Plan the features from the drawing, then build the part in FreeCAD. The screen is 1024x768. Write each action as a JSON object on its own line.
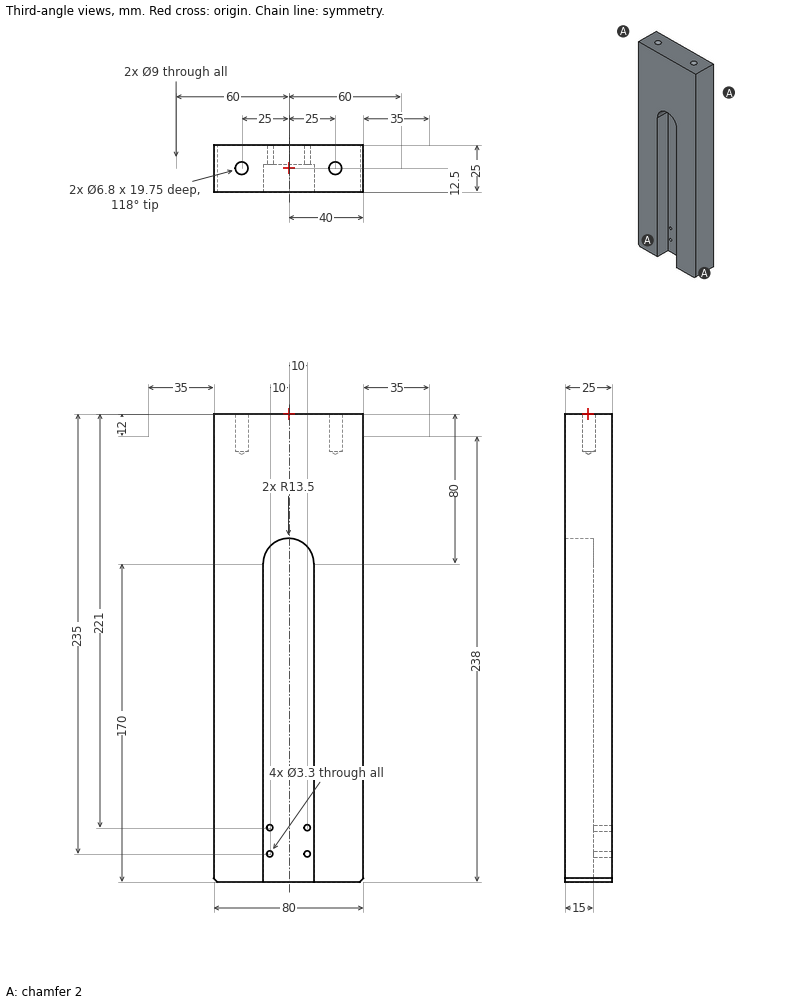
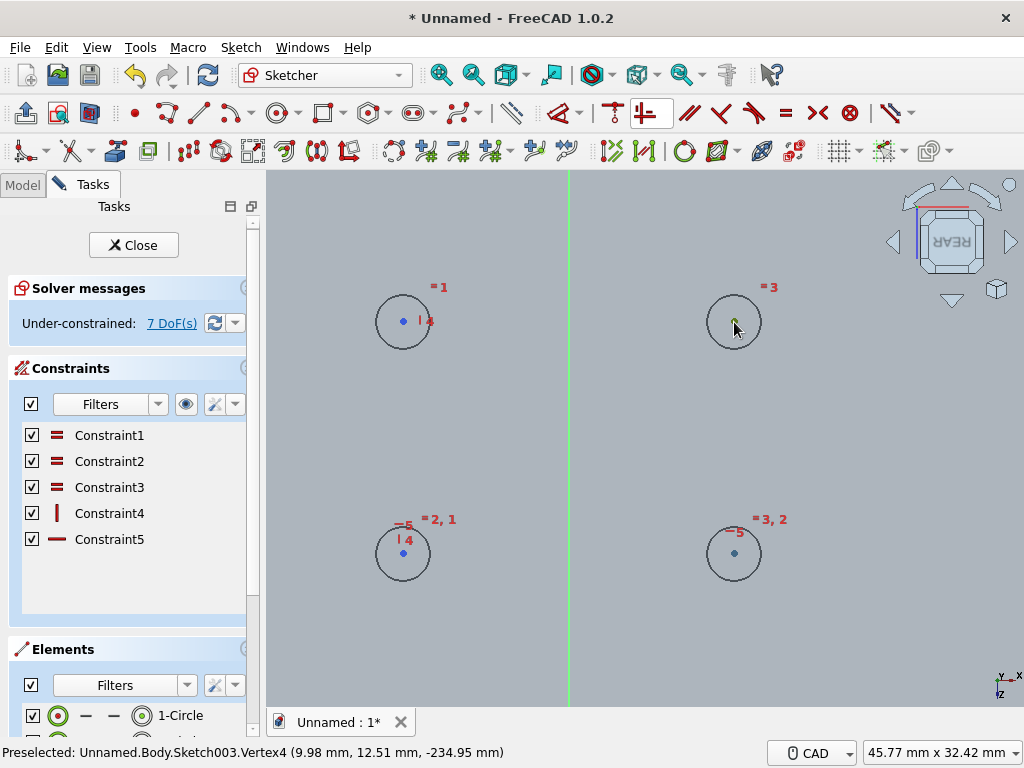
{"action": "left_click", "coordinate": [668, 114]}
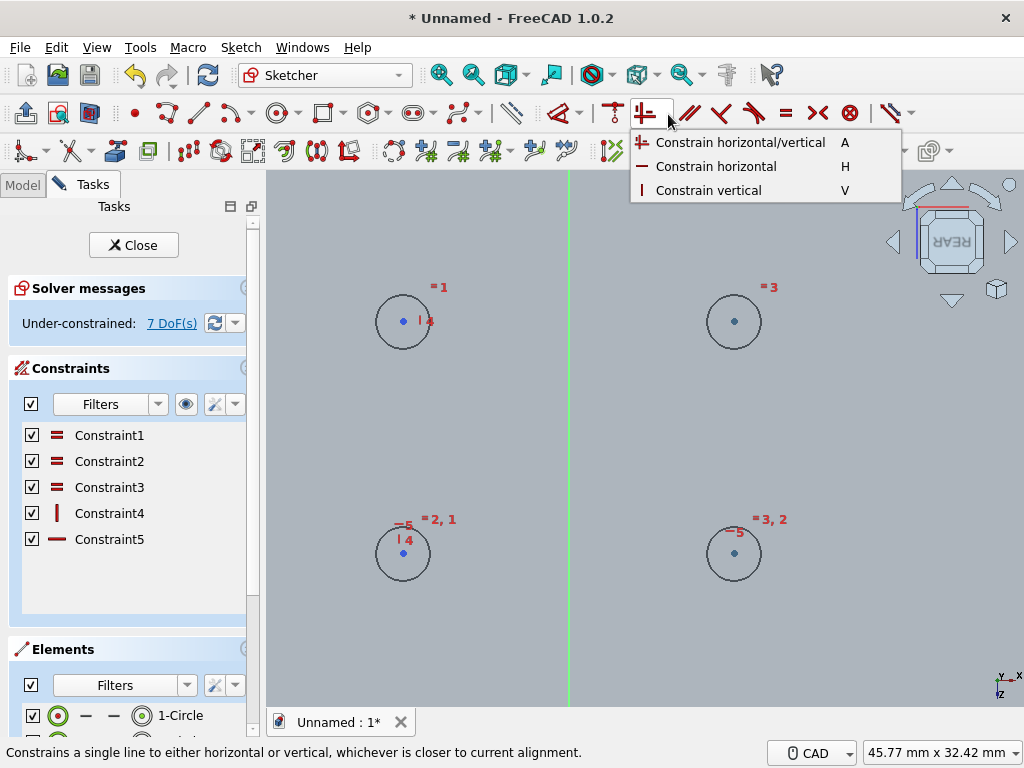
{"action": "left_click", "coordinate": [766, 190]}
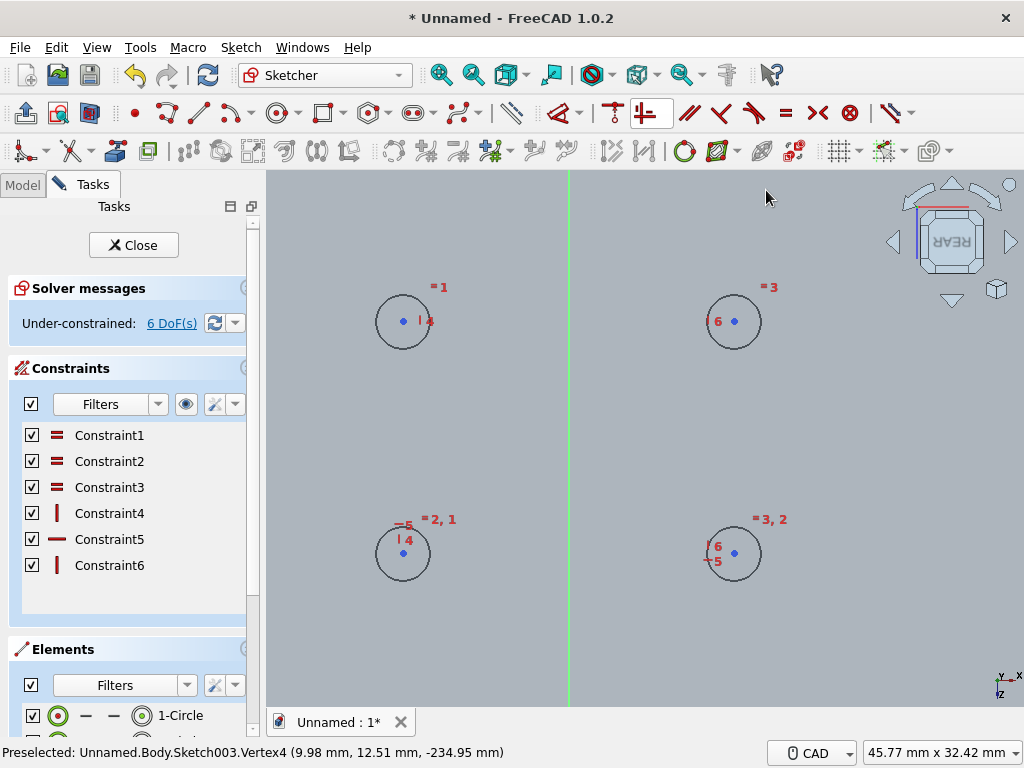
{"action": "left_click", "coordinate": [403, 322]}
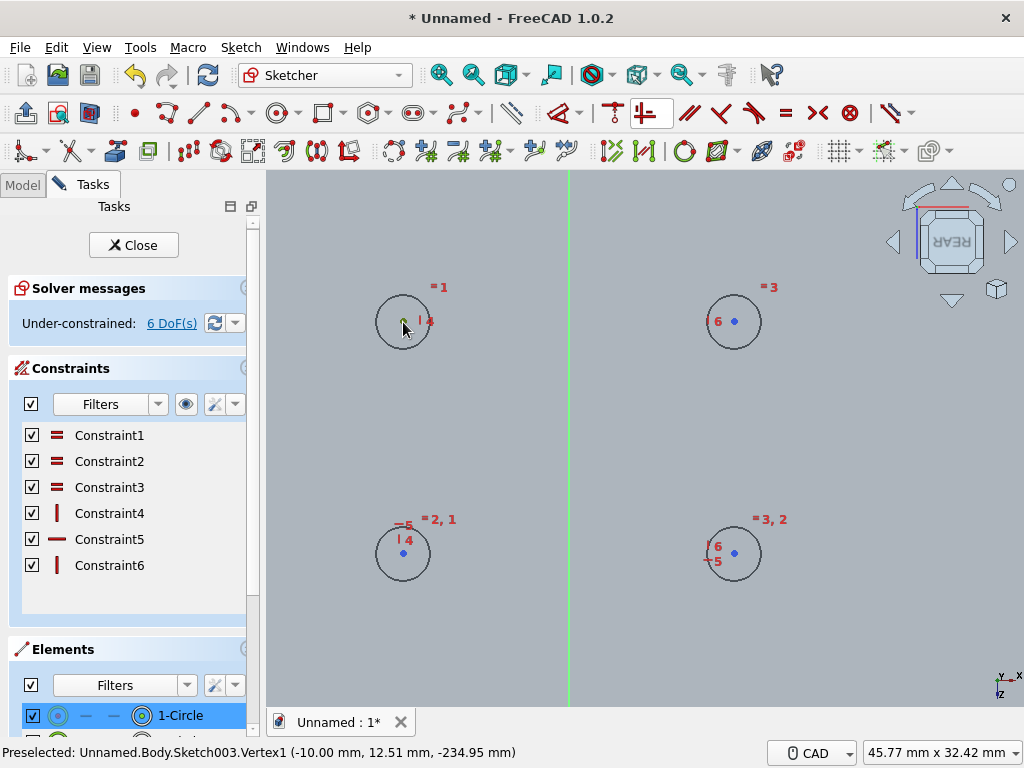
{"action": "left_click", "coordinate": [734, 322]}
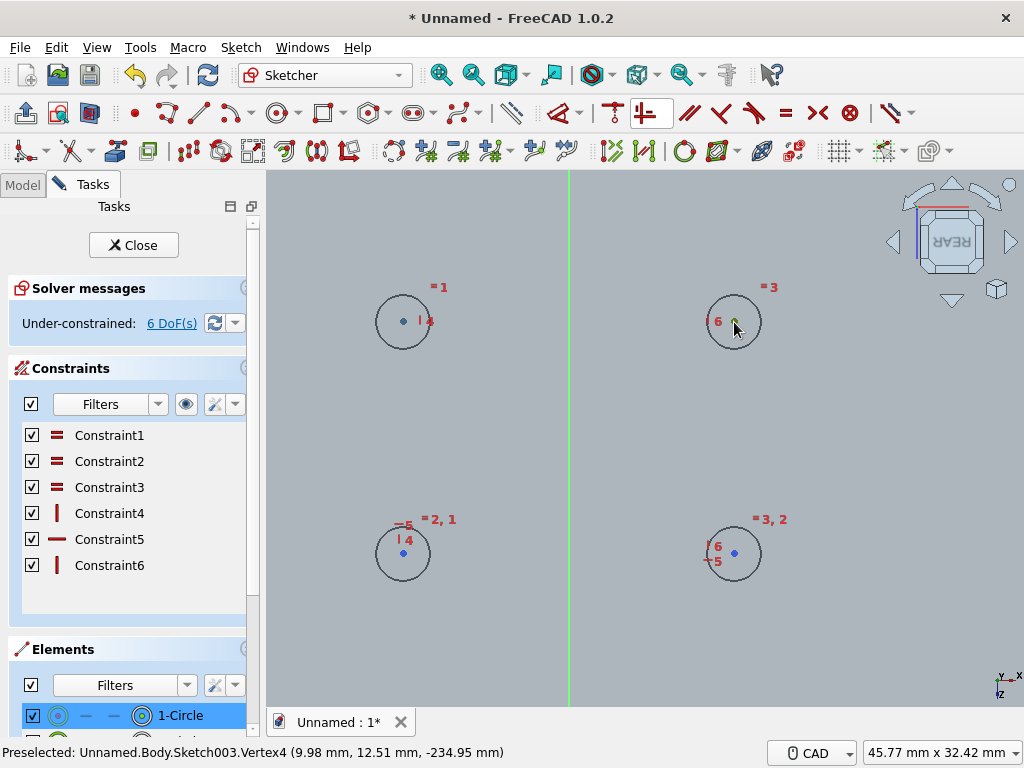
{"action": "left_click", "coordinate": [668, 114]}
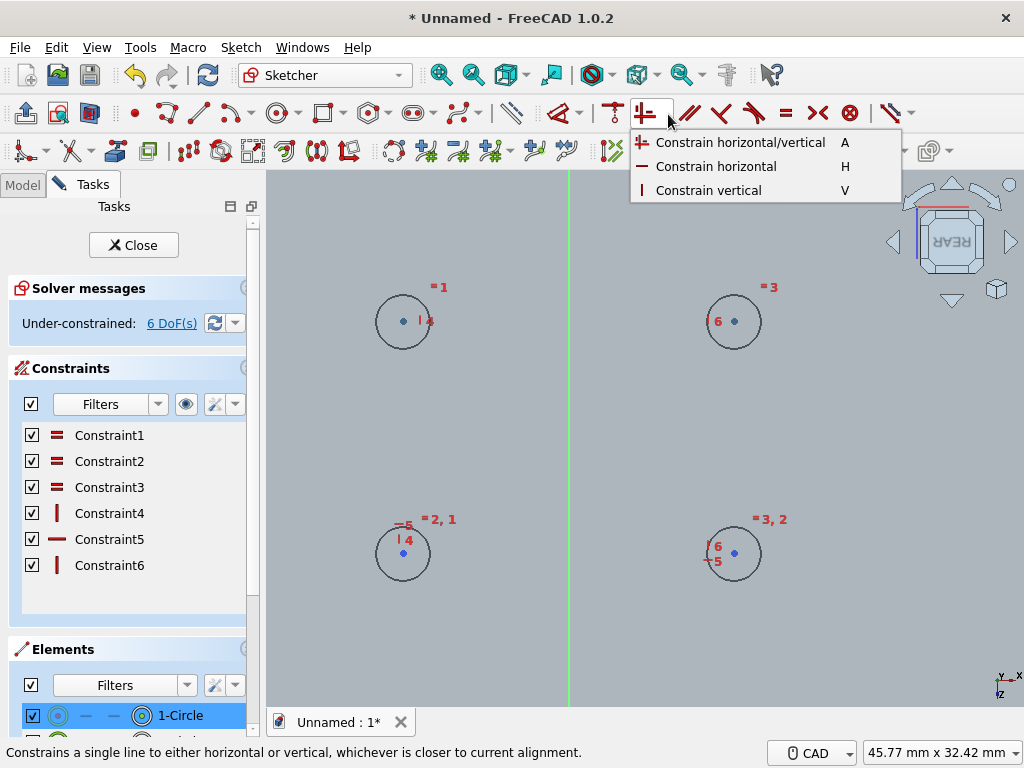
{"action": "left_click", "coordinate": [766, 166]}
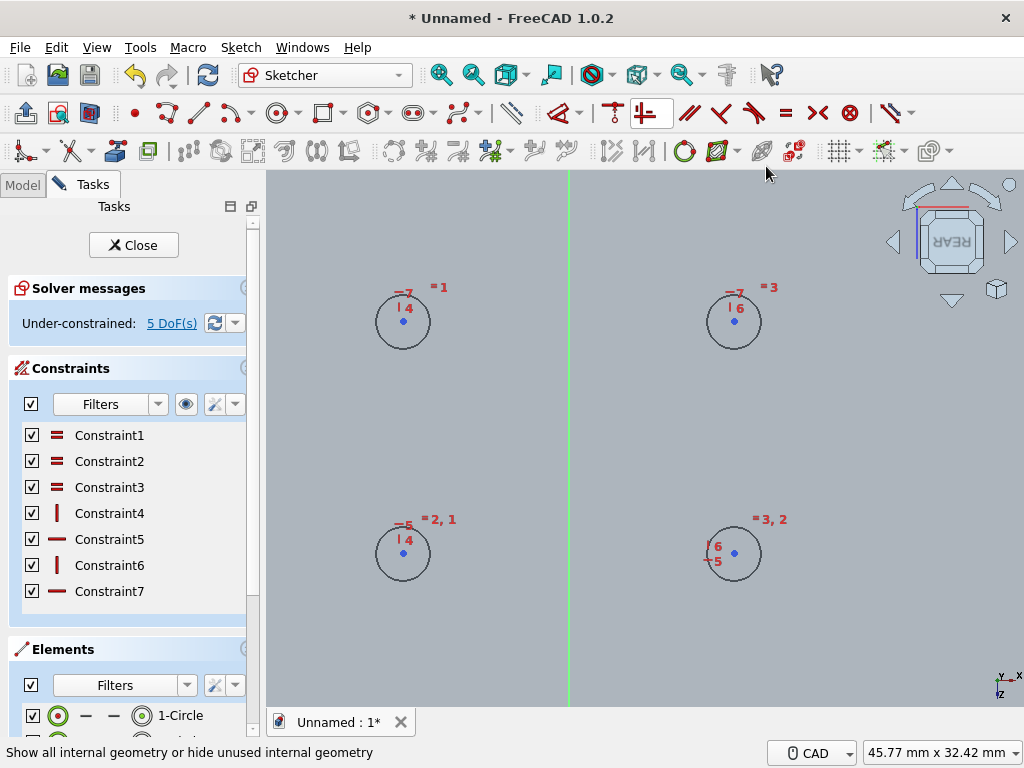
{"action": "left_click", "coordinate": [558, 114]}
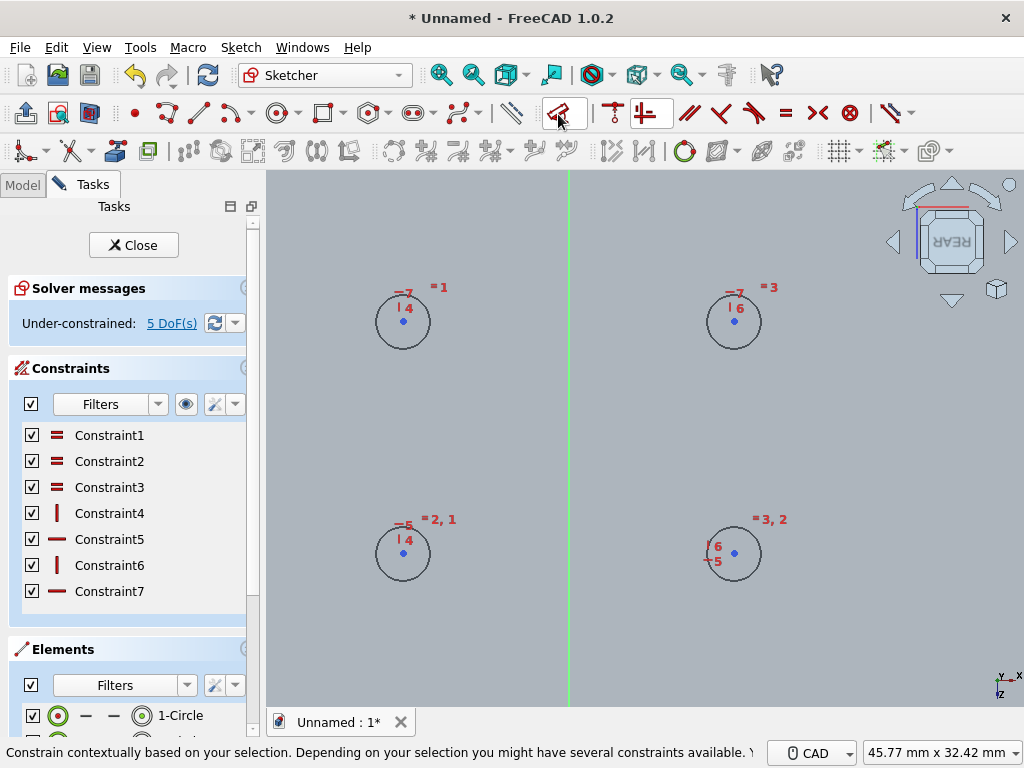
{"action": "left_click", "coordinate": [422, 303]}
{"action": "left_click", "coordinate": [445, 280]}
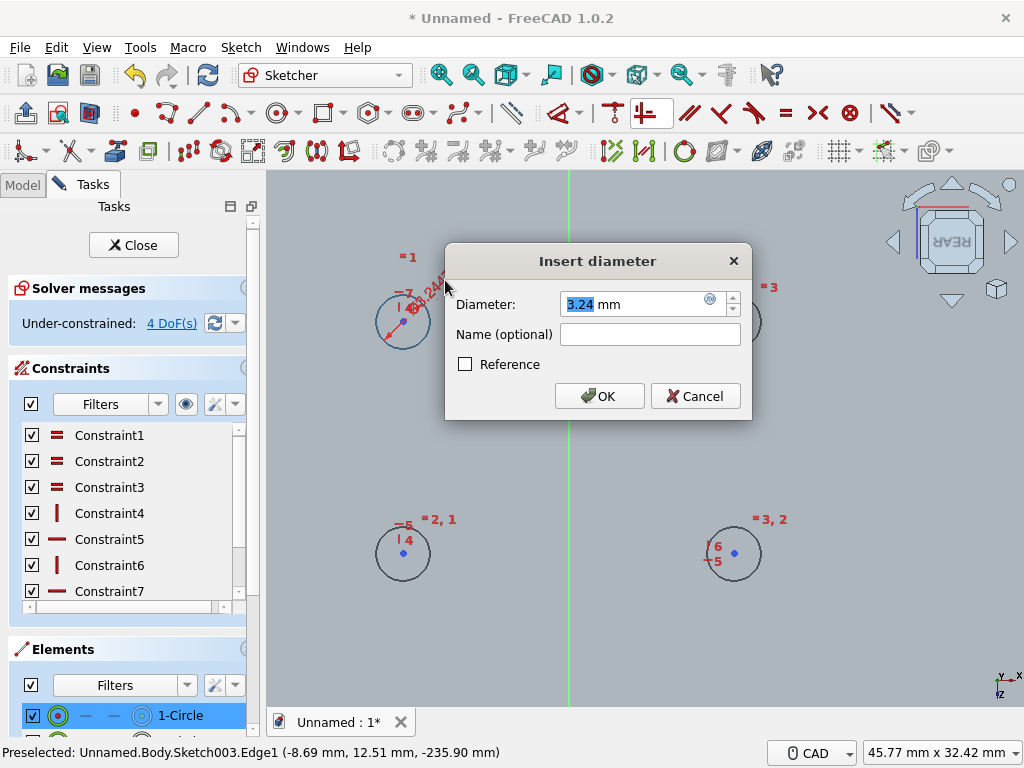
{"action": "type", "text": "3.3"}
{"action": "key", "text": "Return"}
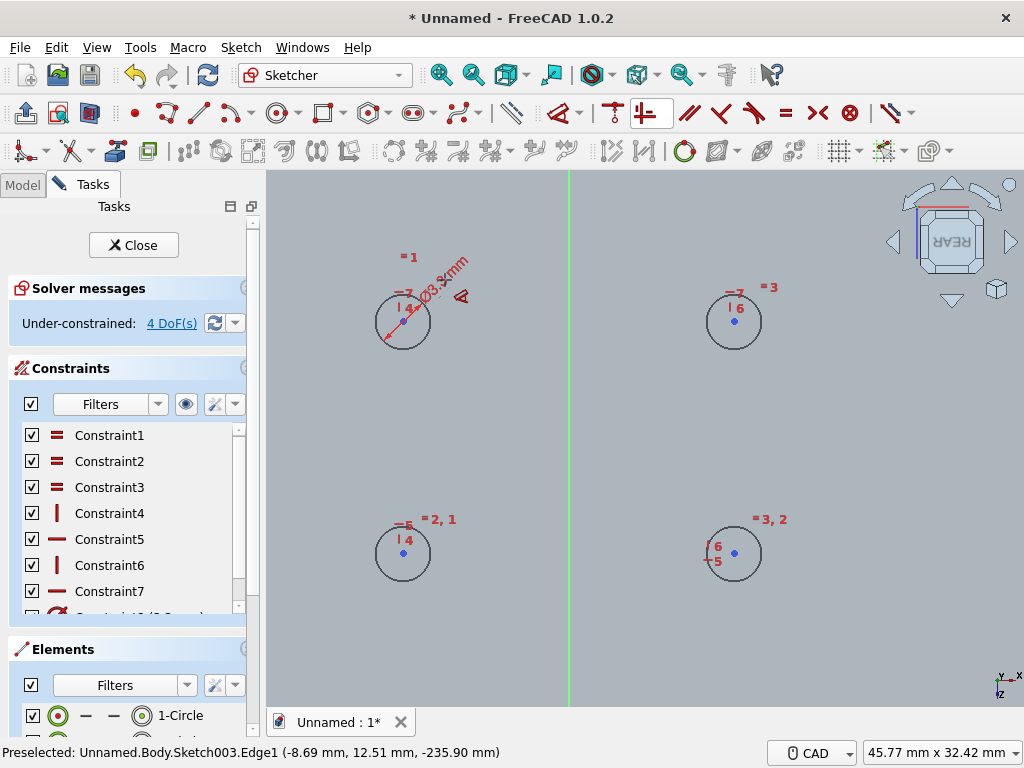
{"action": "left_click", "coordinate": [403, 322]}
{"action": "left_click", "coordinate": [524, 288]}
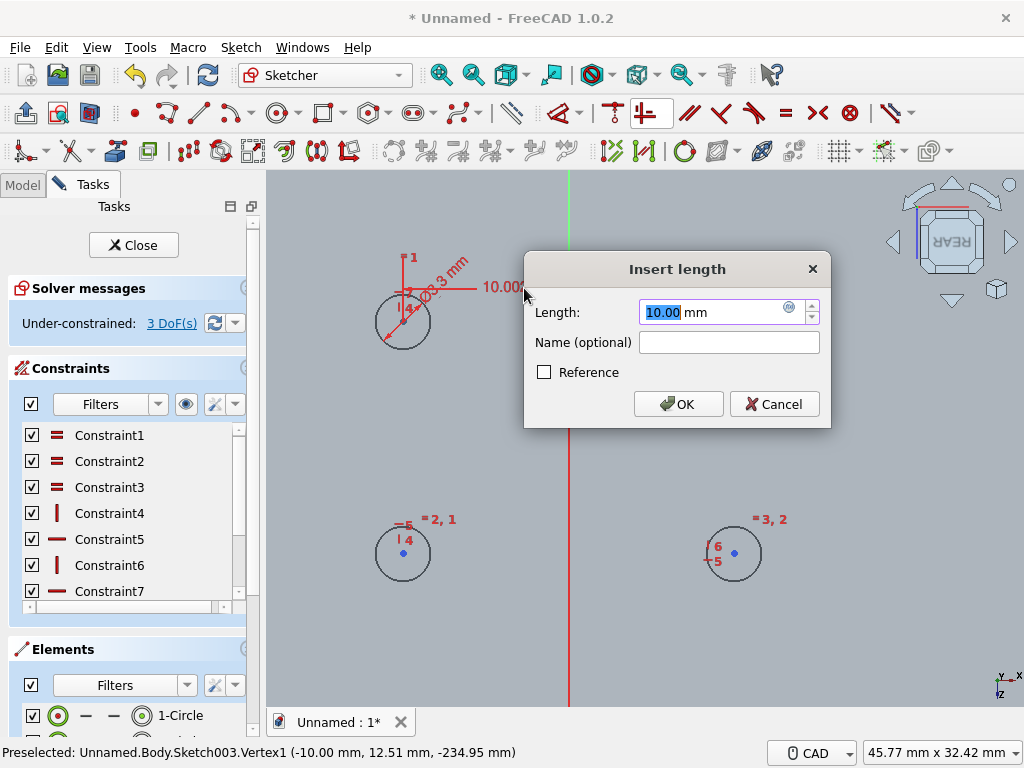
{"action": "type", "text": "10"}
{"action": "key", "text": "Return"}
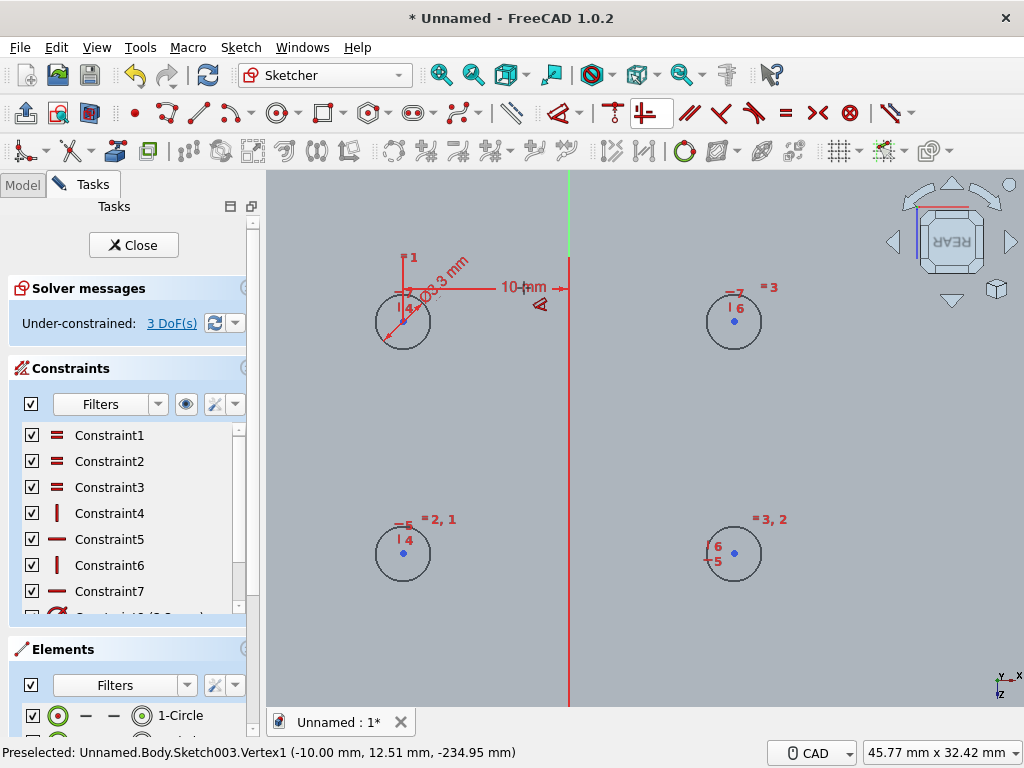
{"action": "left_click", "coordinate": [734, 554]}
{"action": "left_click", "coordinate": [651, 520]}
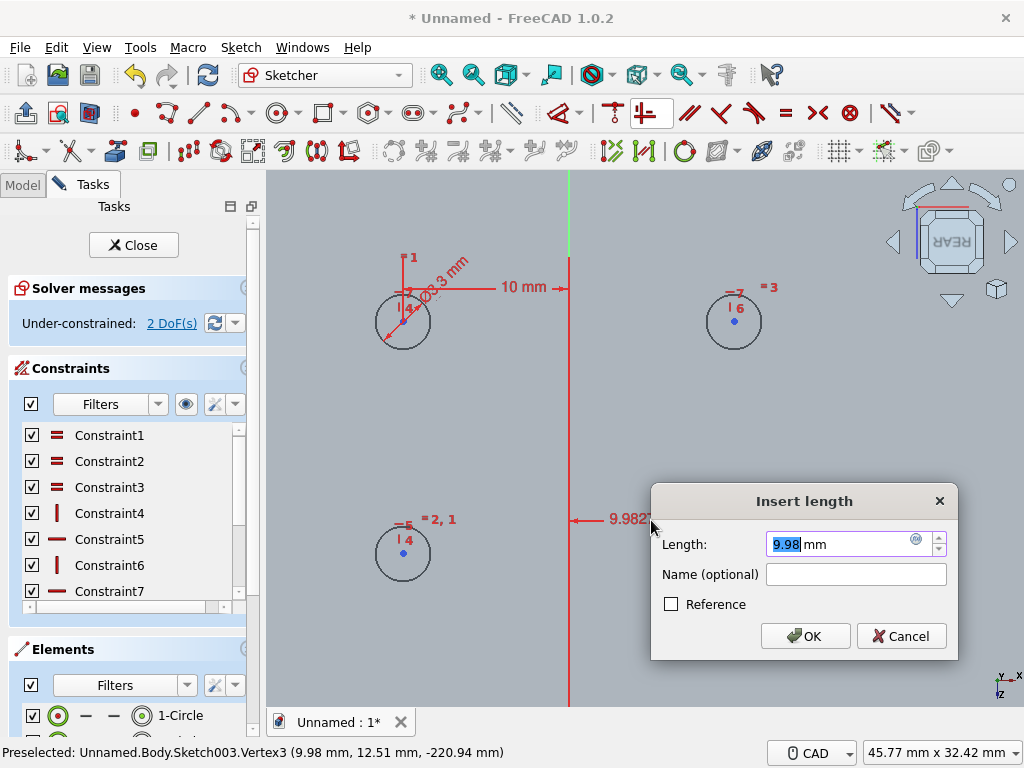
{"action": "type", "text": "10"}
{"action": "key", "text": "Return"}